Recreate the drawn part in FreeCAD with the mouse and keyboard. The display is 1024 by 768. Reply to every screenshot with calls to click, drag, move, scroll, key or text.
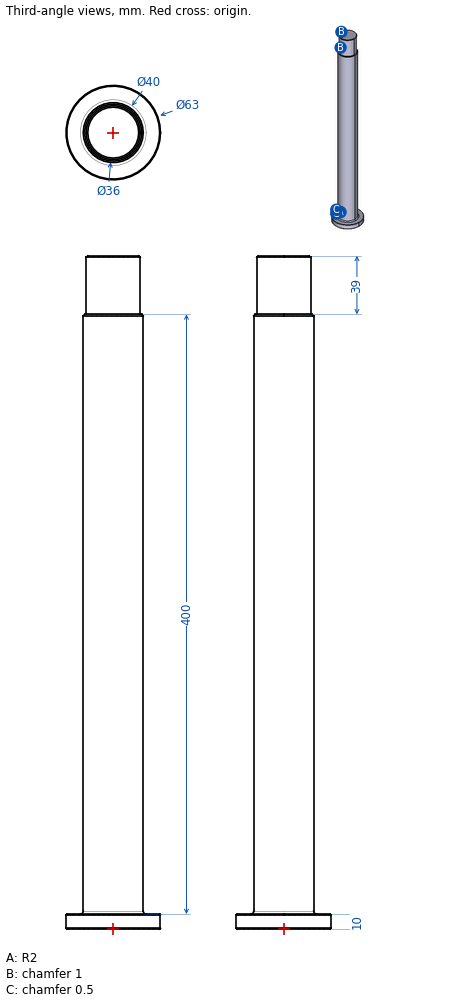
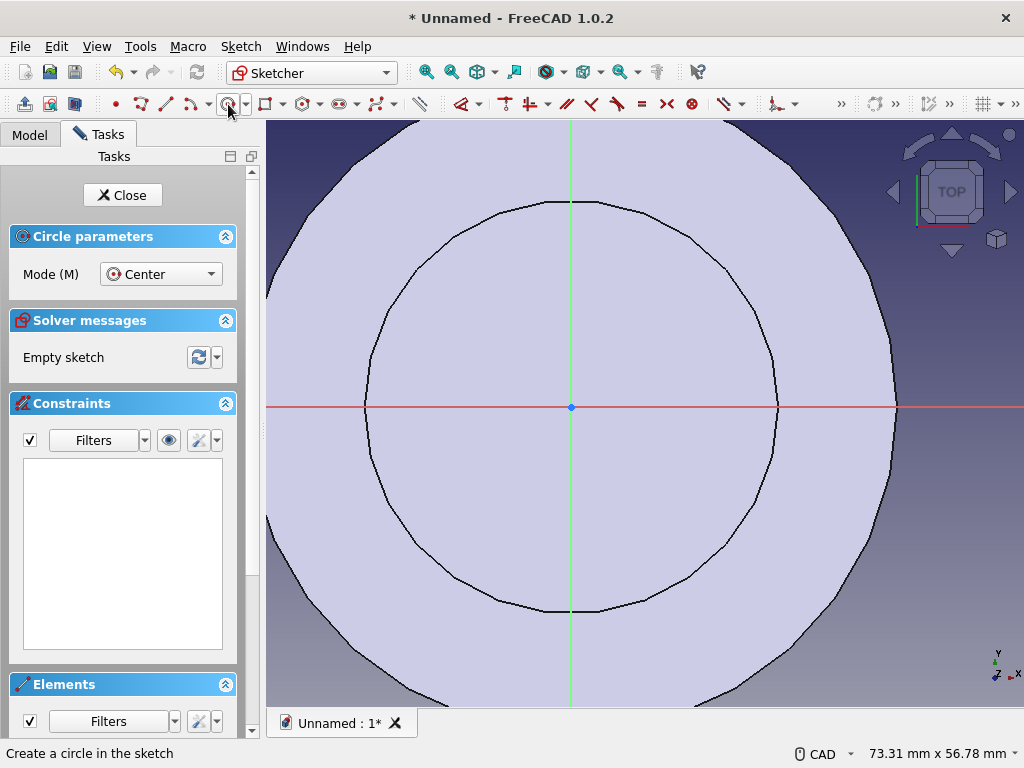
click(571, 407)
move(703, 276)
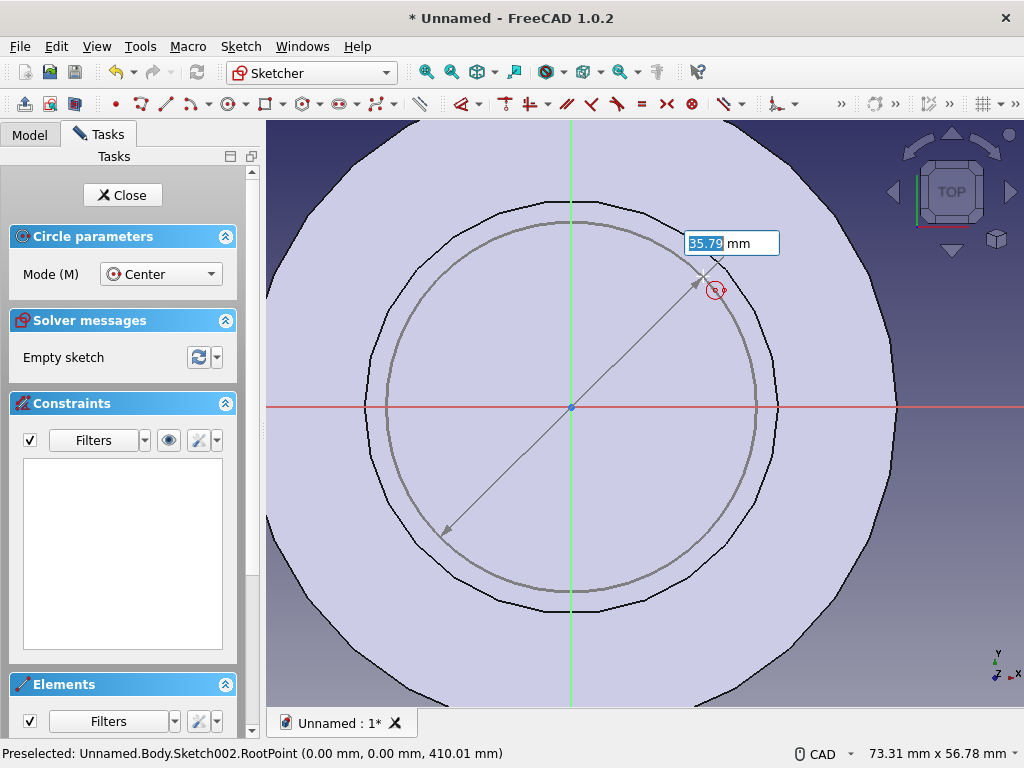
text(36)
key(Return)
key(Escape)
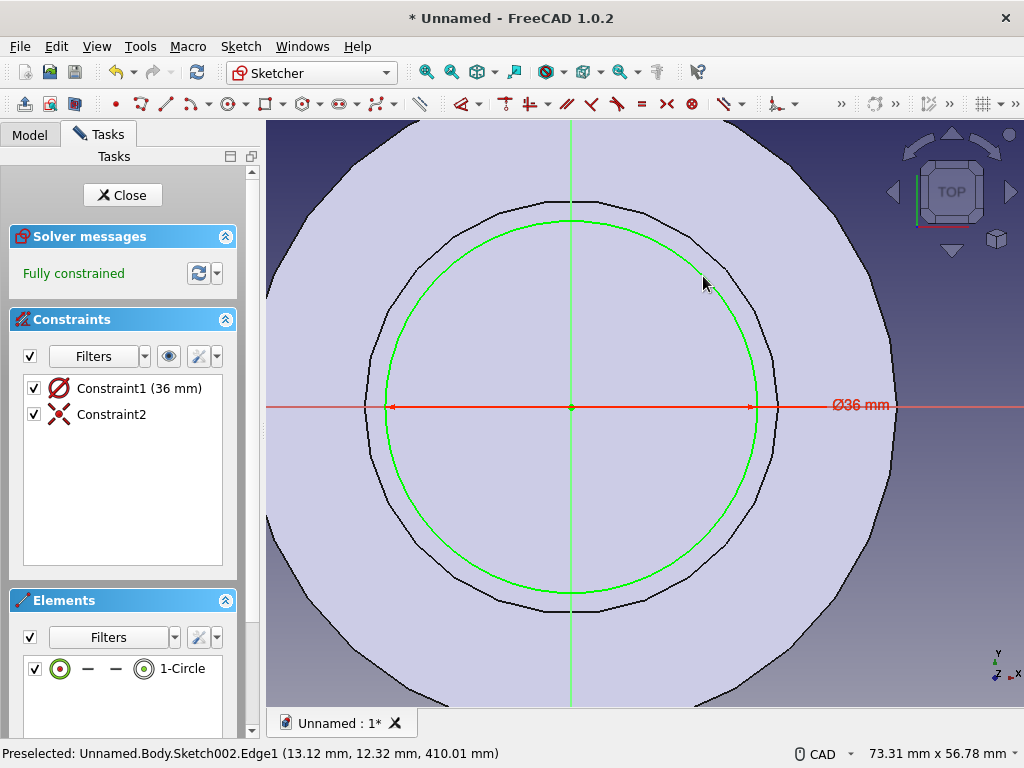
click(123, 195)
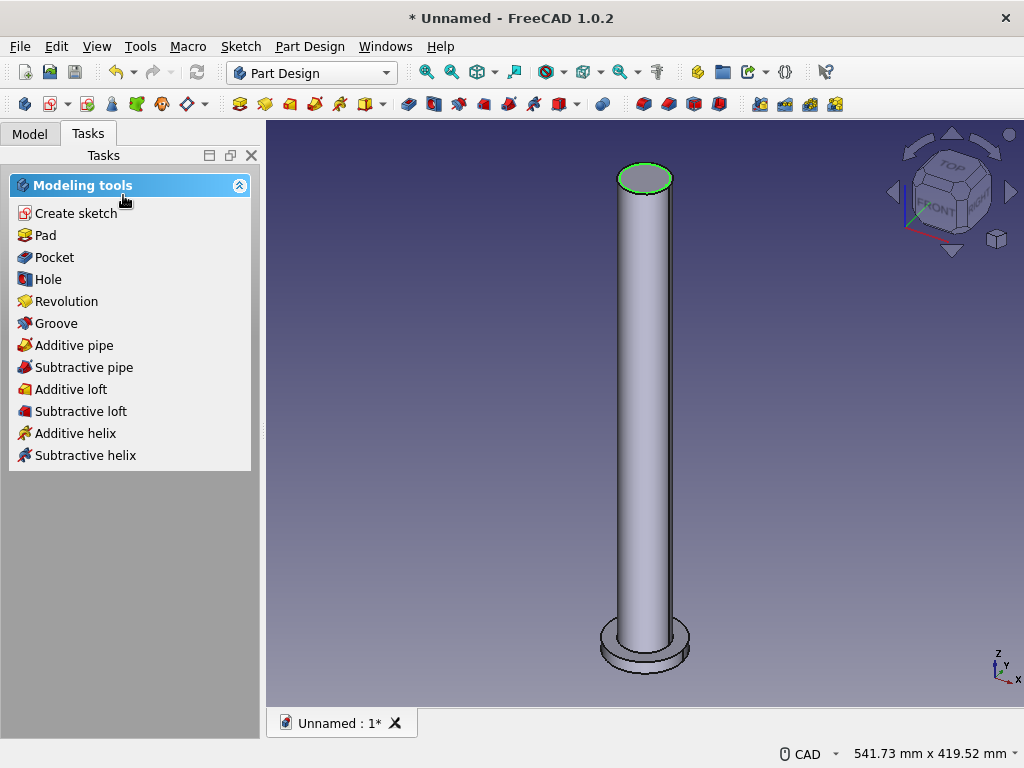
click(240, 104)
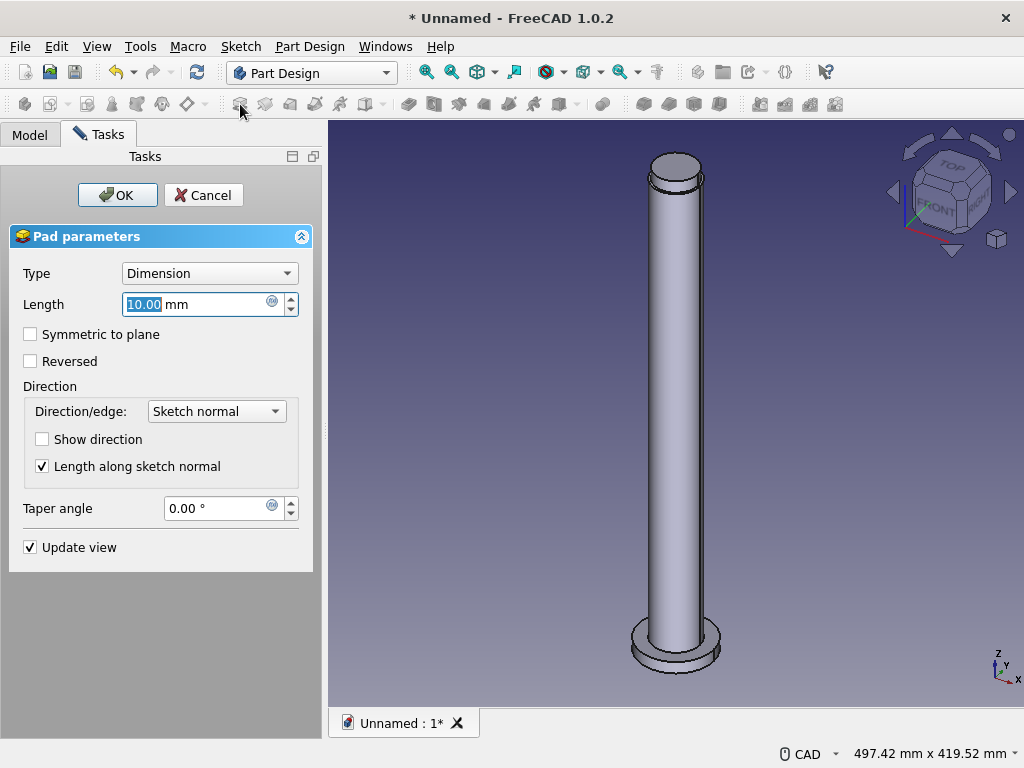
text(39)
key(Tab)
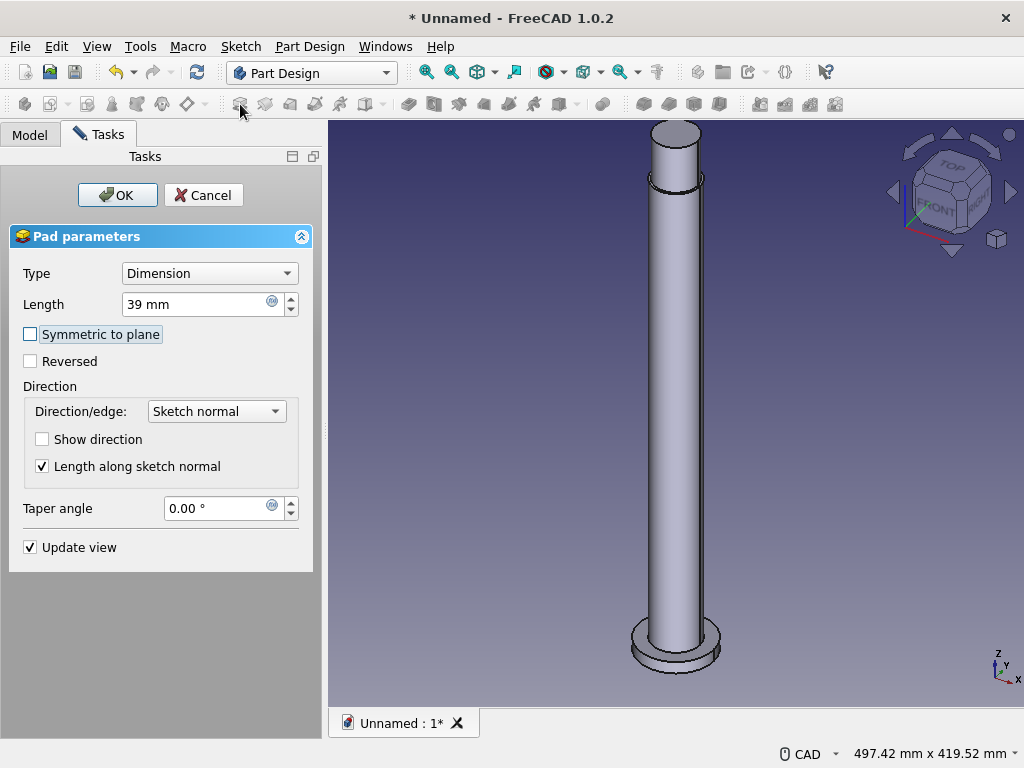
click(118, 195)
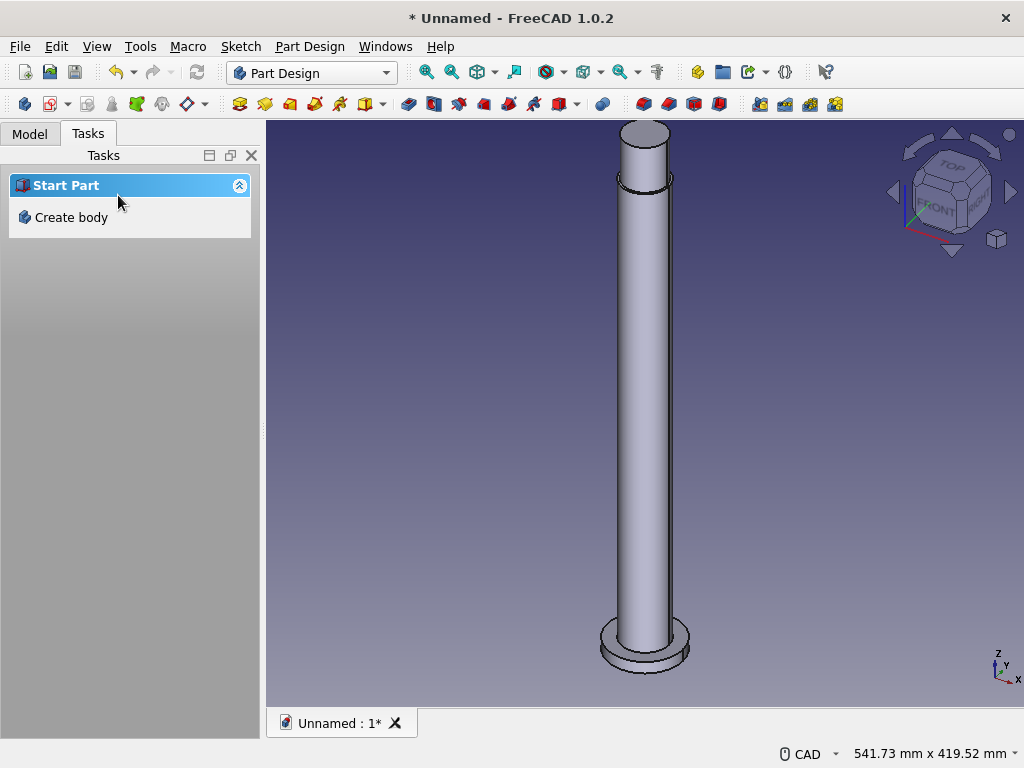
click(427, 72)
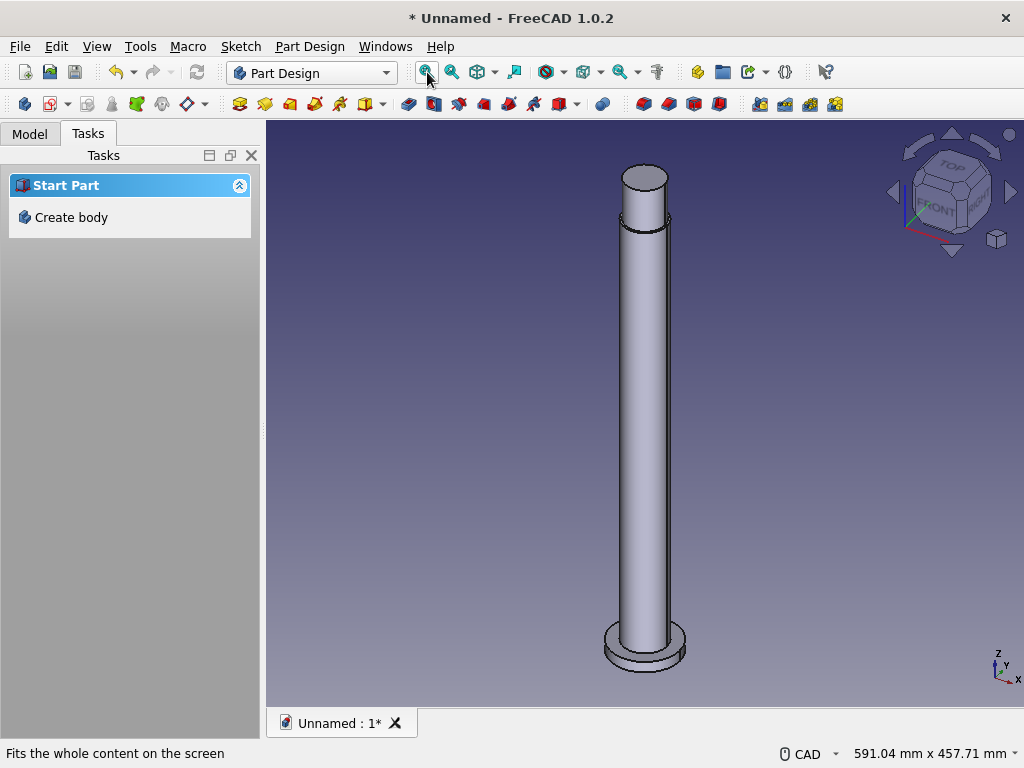
key(0)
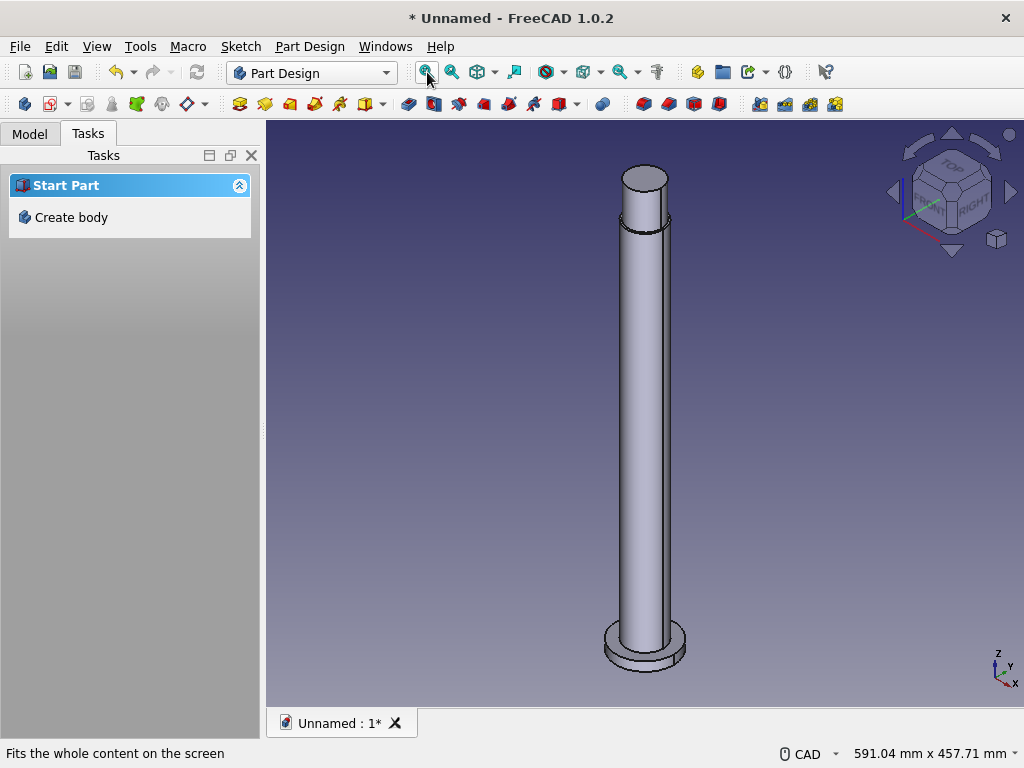
click(622, 644)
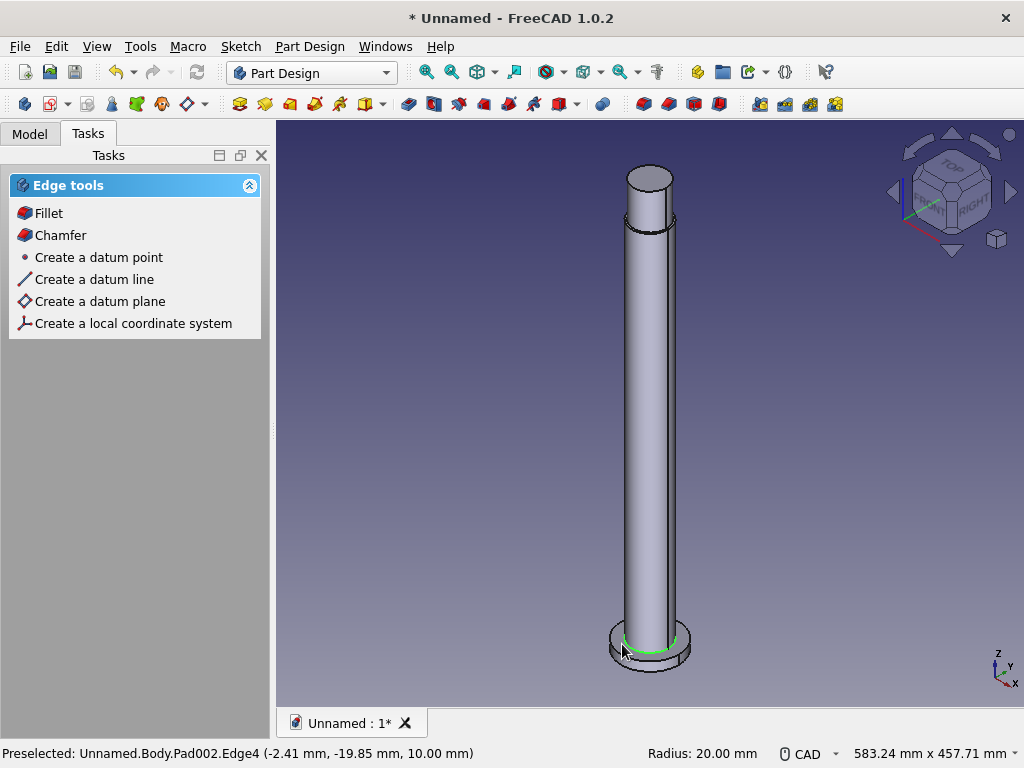
click(644, 104)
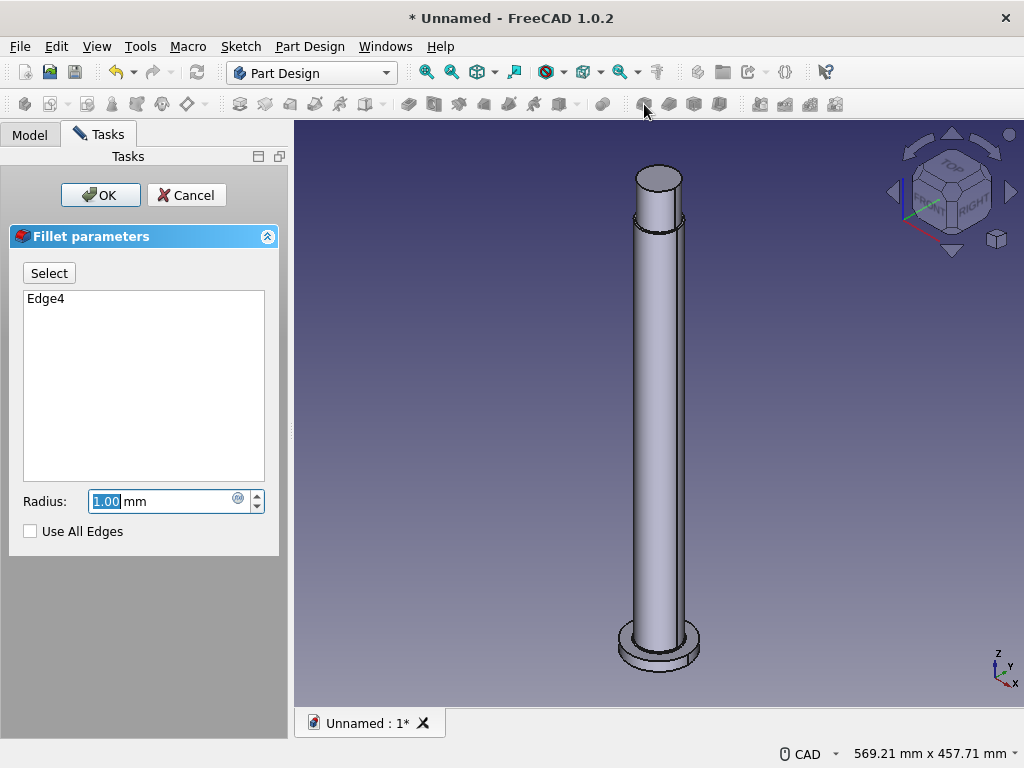
text(2)
key(Tab)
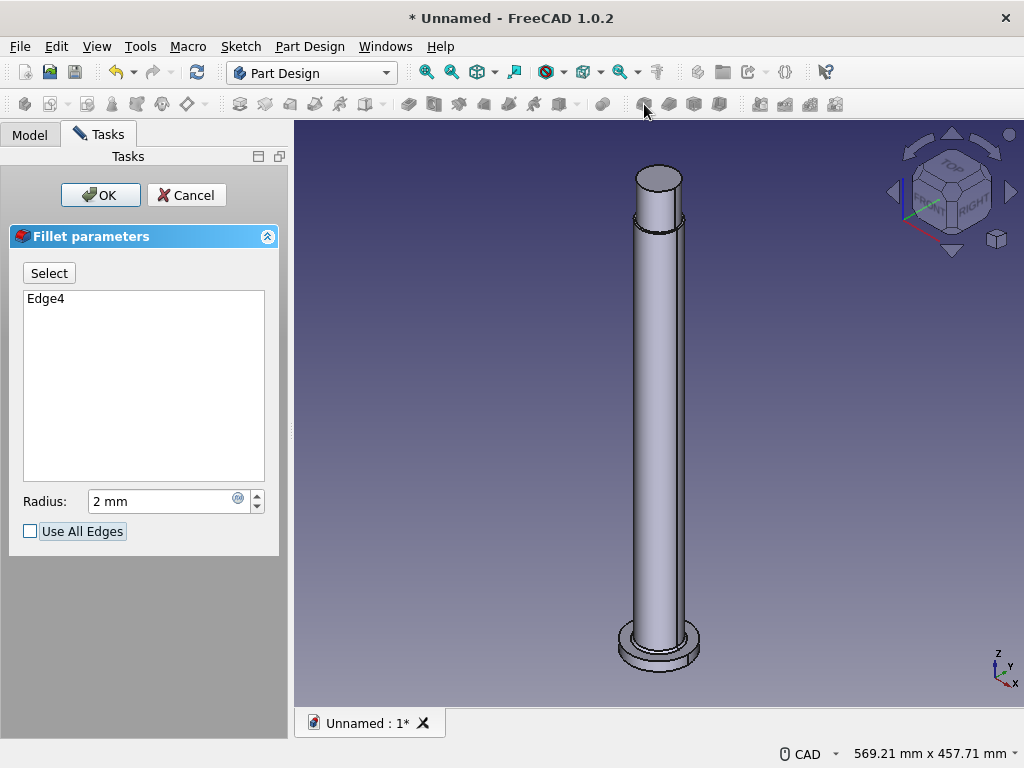
click(101, 195)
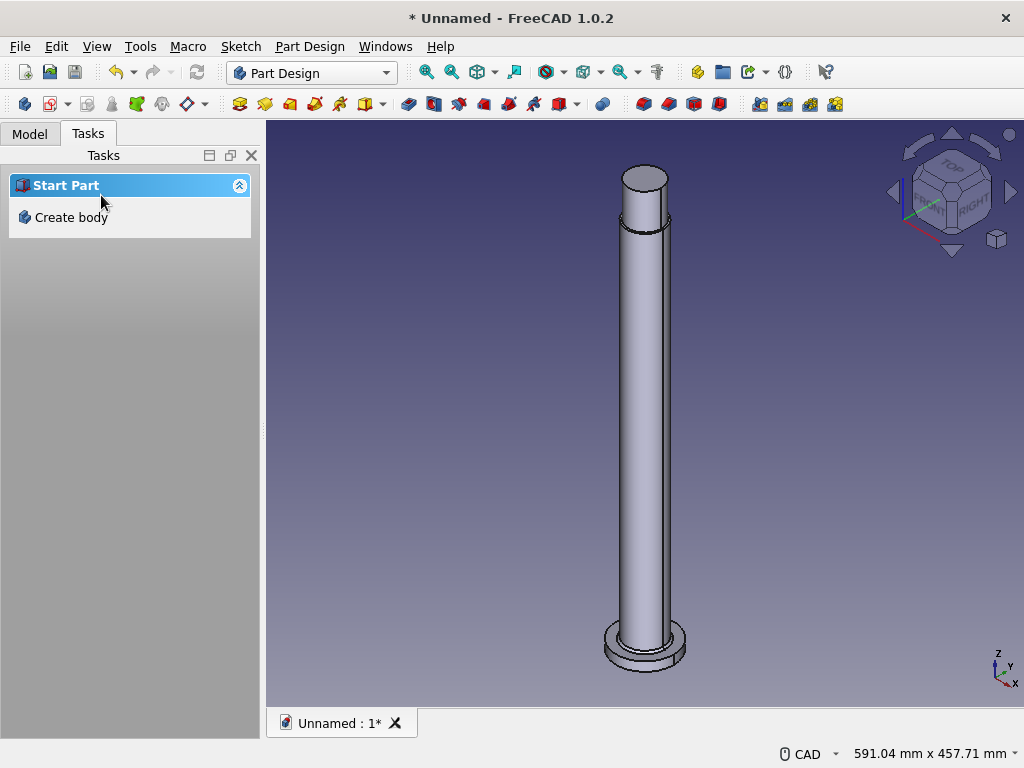
click(622, 175)